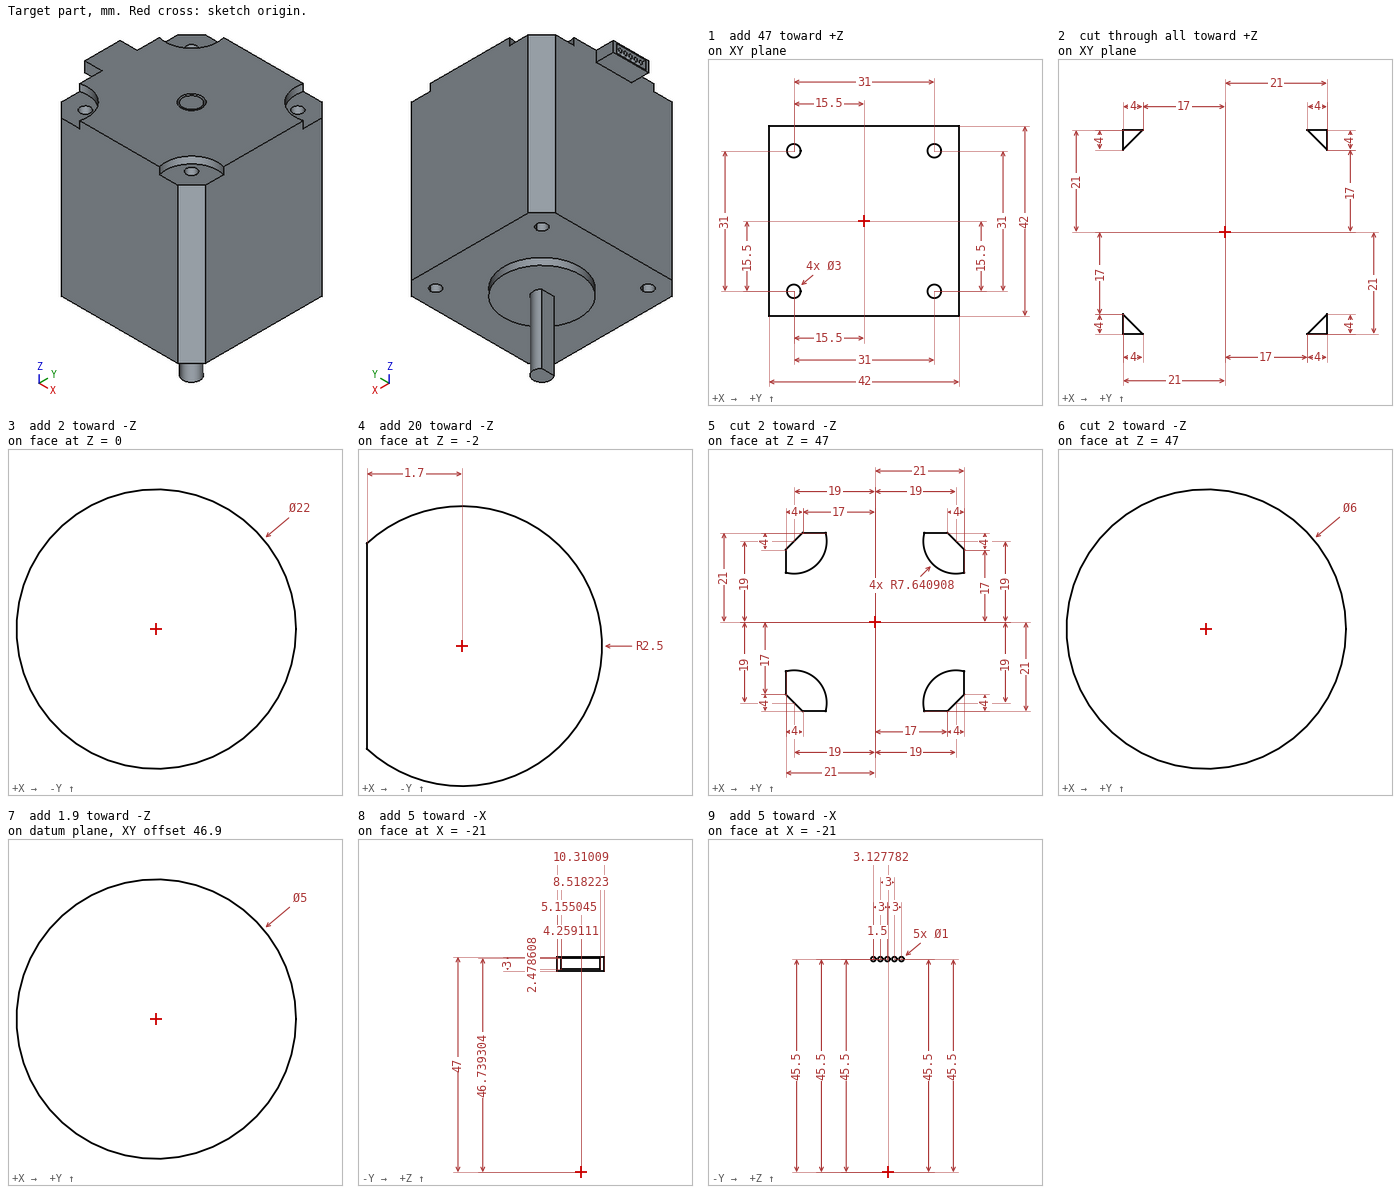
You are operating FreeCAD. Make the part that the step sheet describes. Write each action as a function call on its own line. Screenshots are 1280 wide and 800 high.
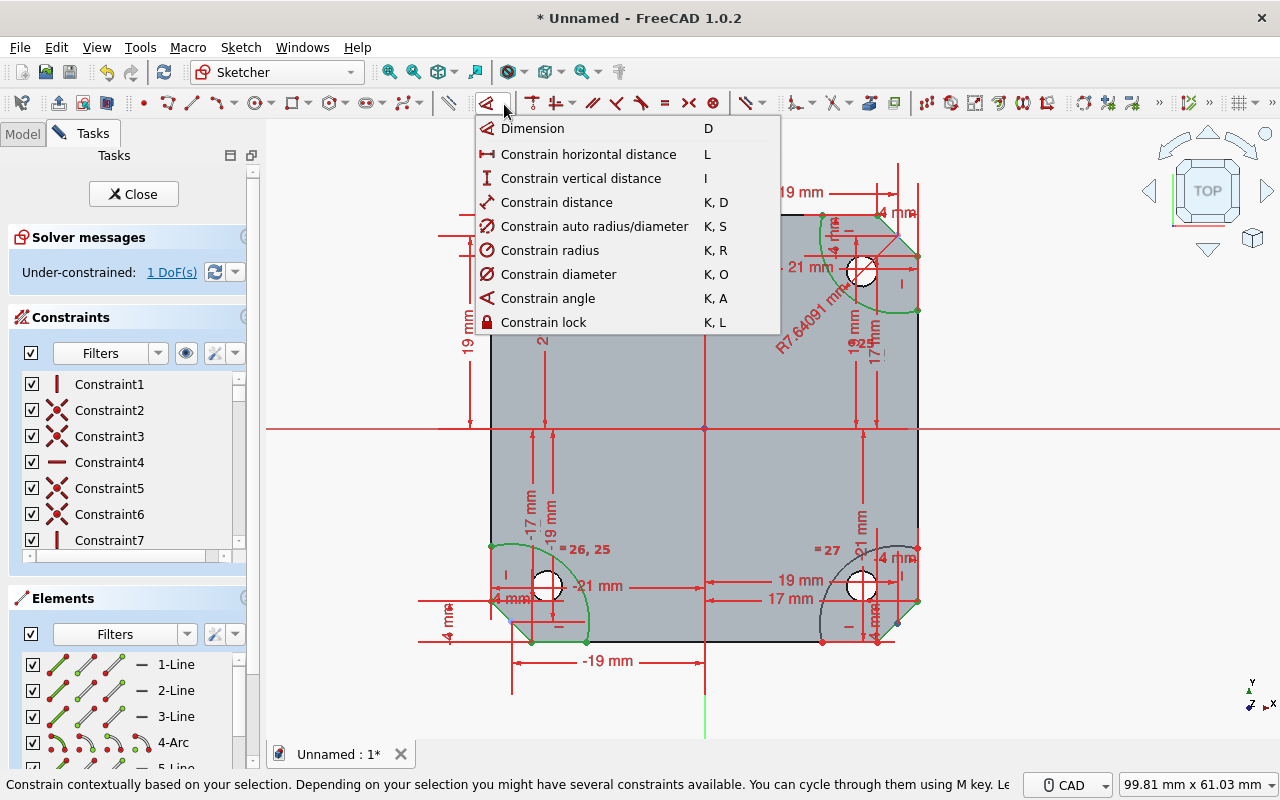
click(628, 178)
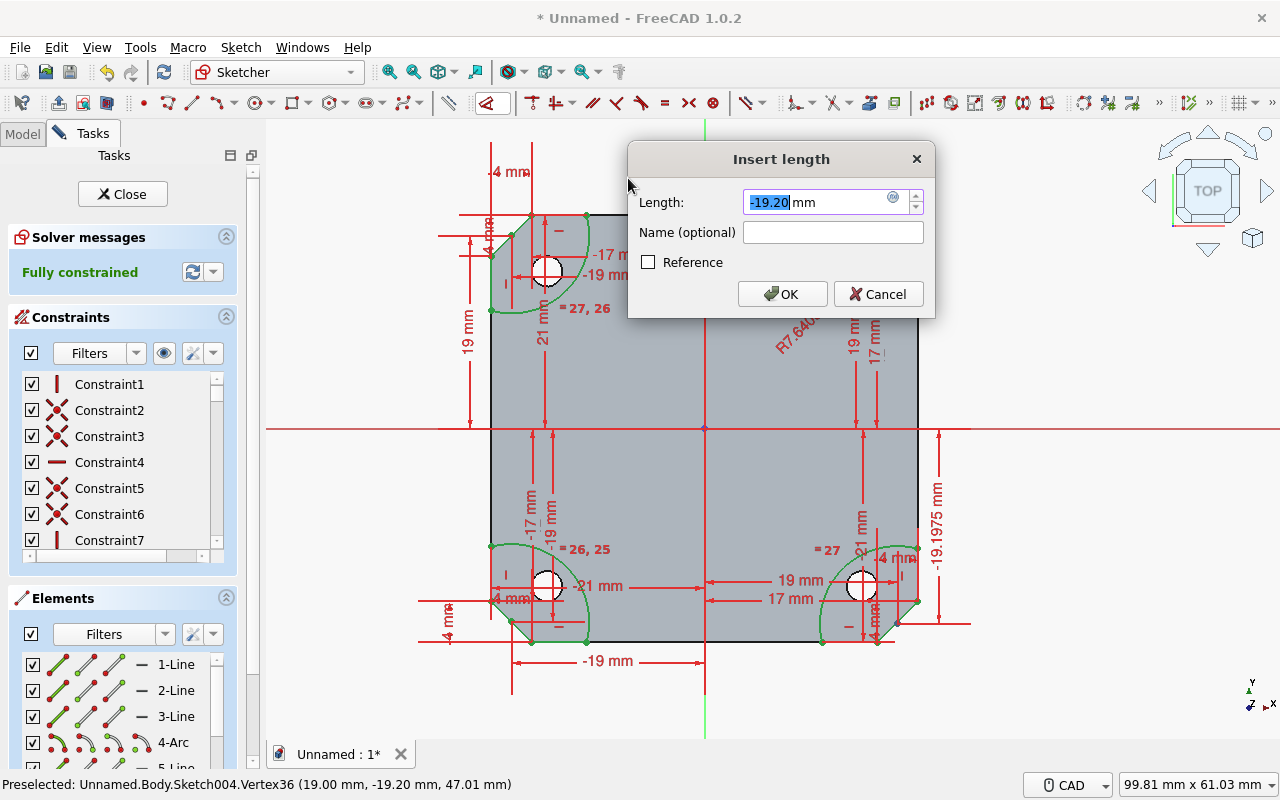
text(-19)
key(Return)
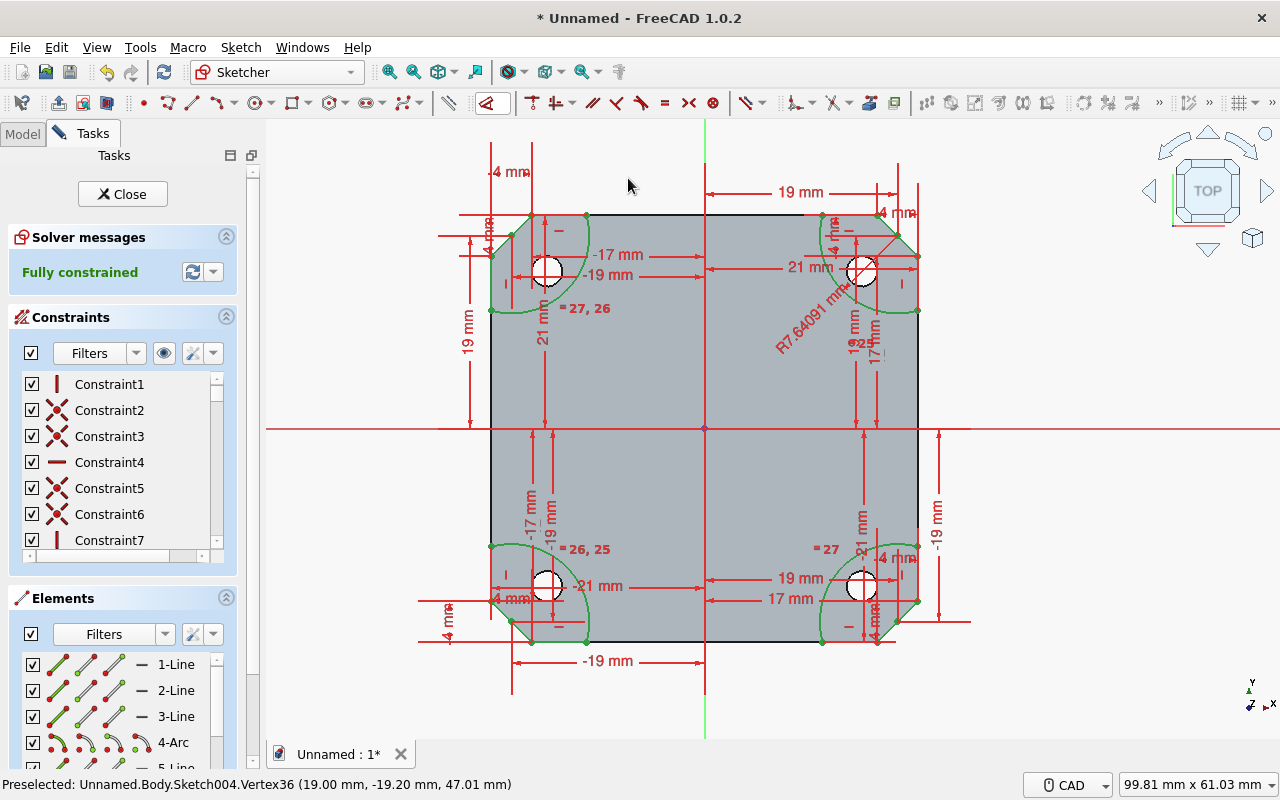
click(123, 194)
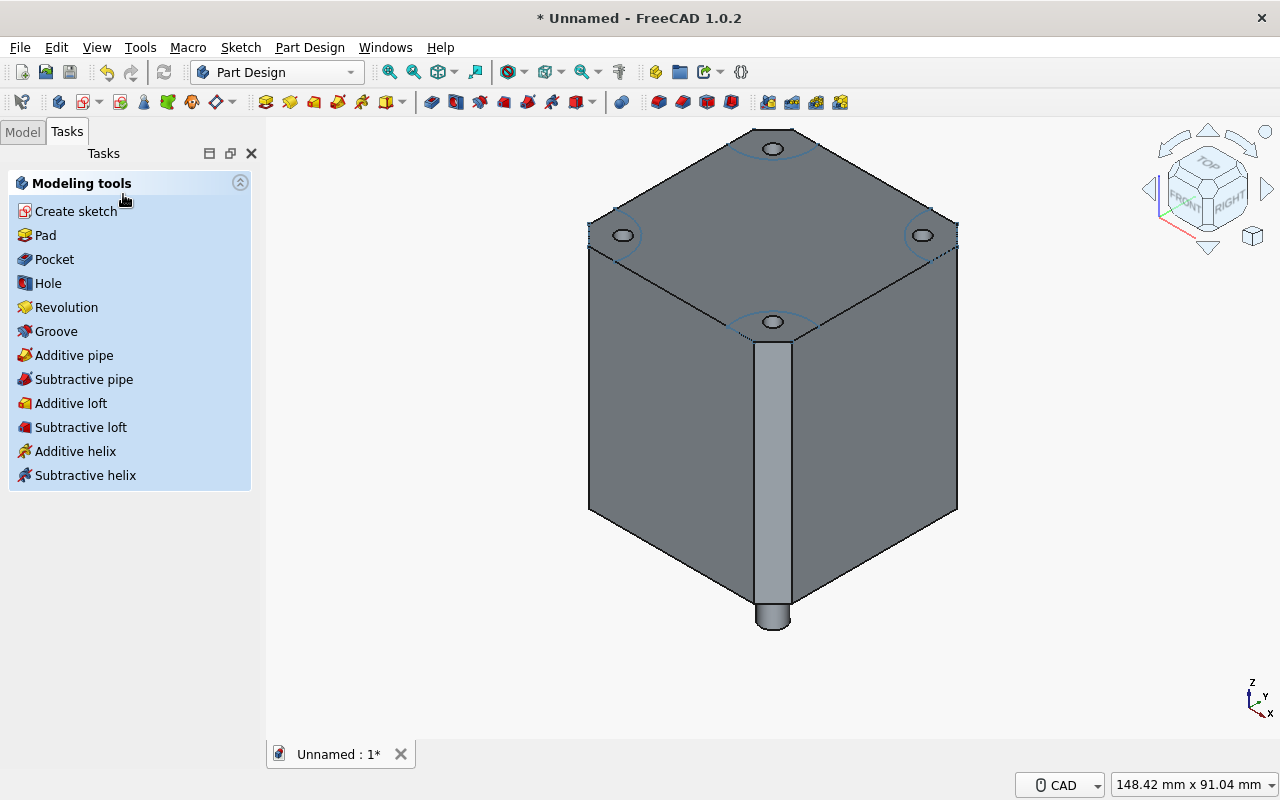
click(432, 102)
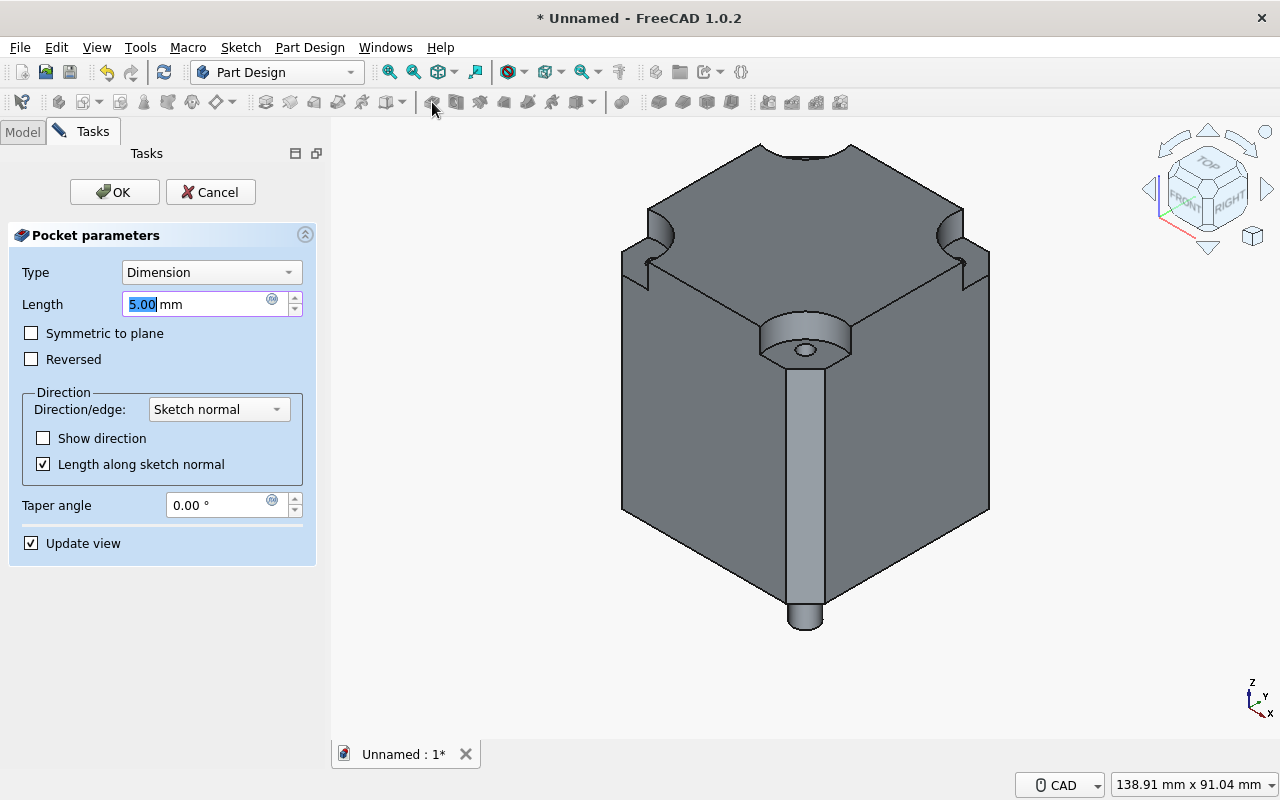
text(2)
key(Tab)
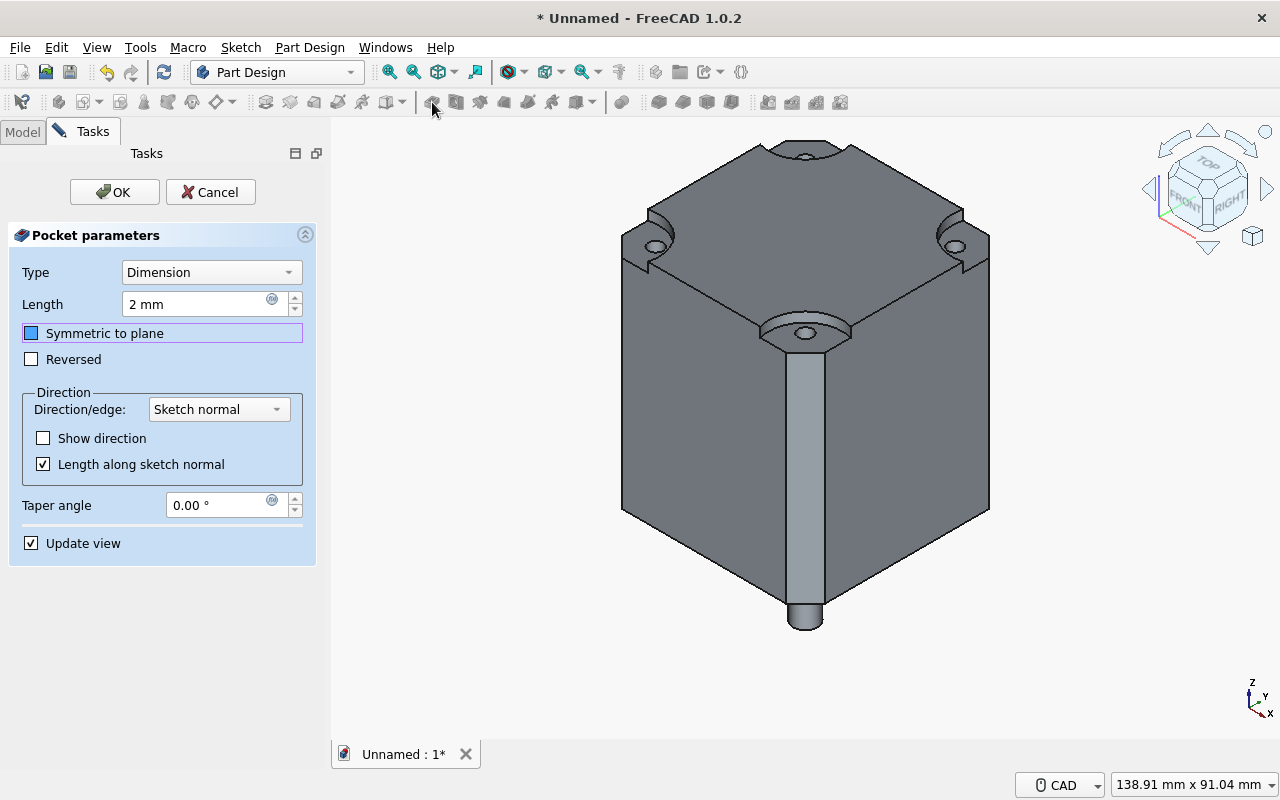
click(115, 192)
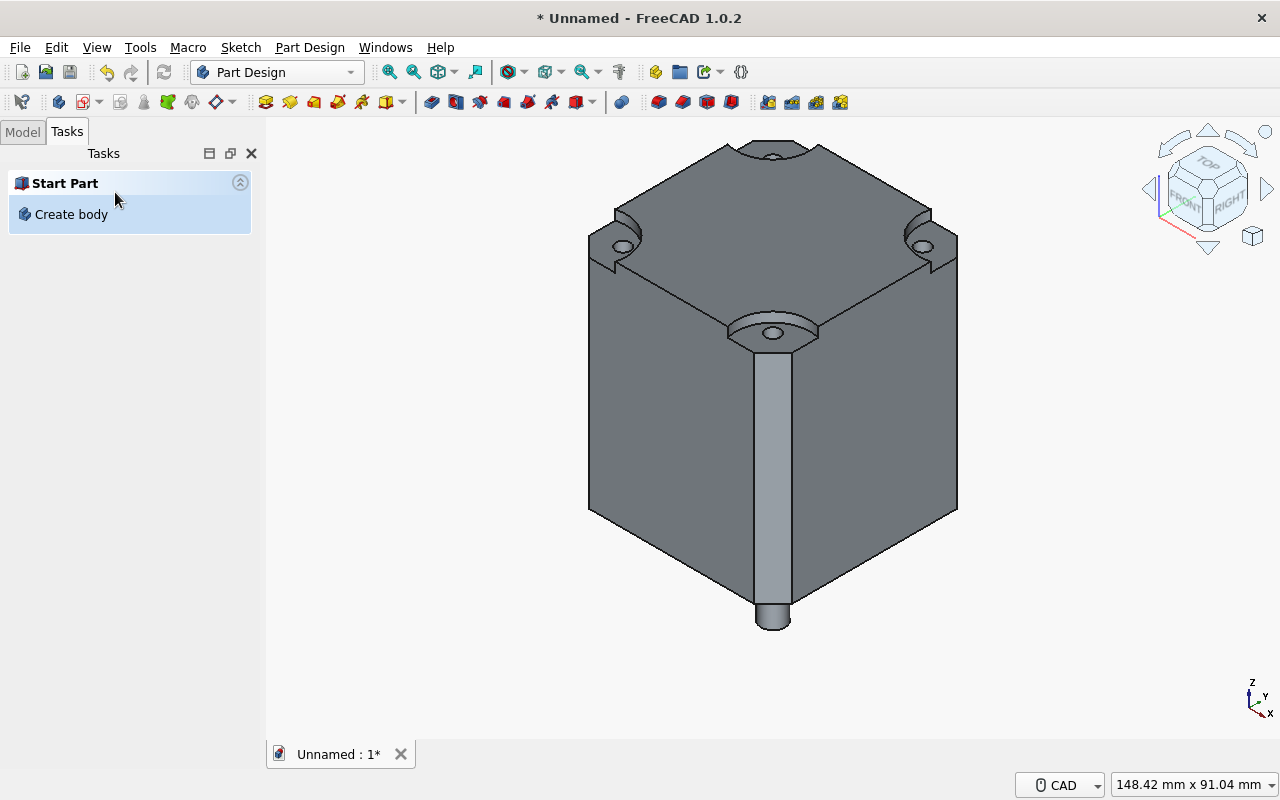
click(773, 235)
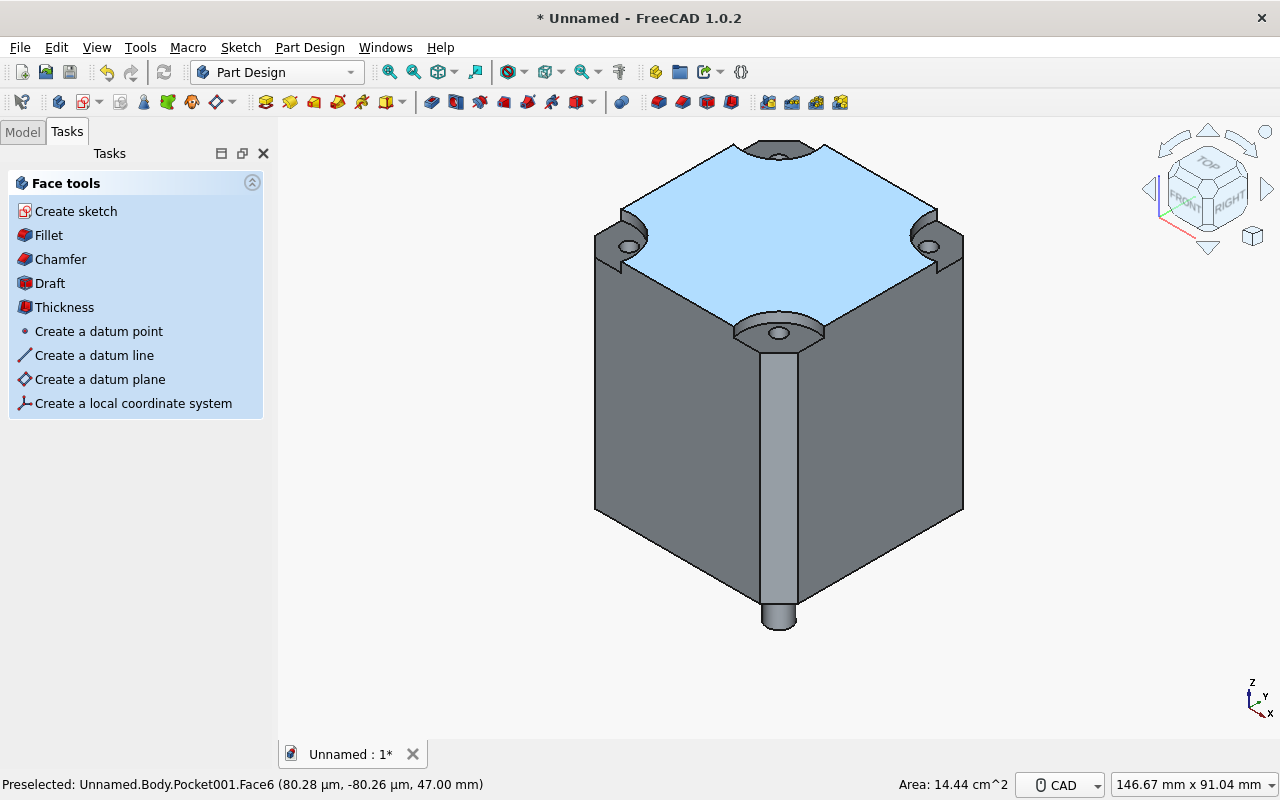
click(84, 102)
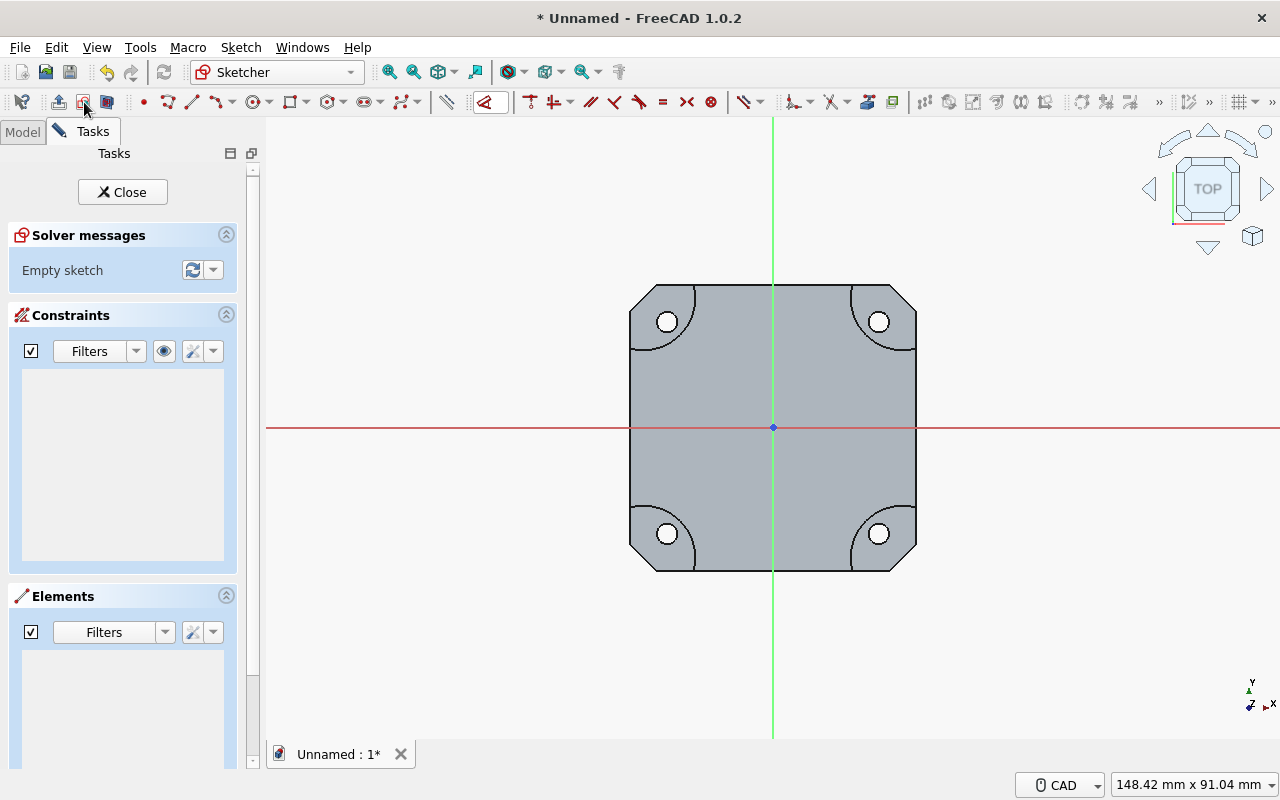
scroll(782, 428, up, 11)